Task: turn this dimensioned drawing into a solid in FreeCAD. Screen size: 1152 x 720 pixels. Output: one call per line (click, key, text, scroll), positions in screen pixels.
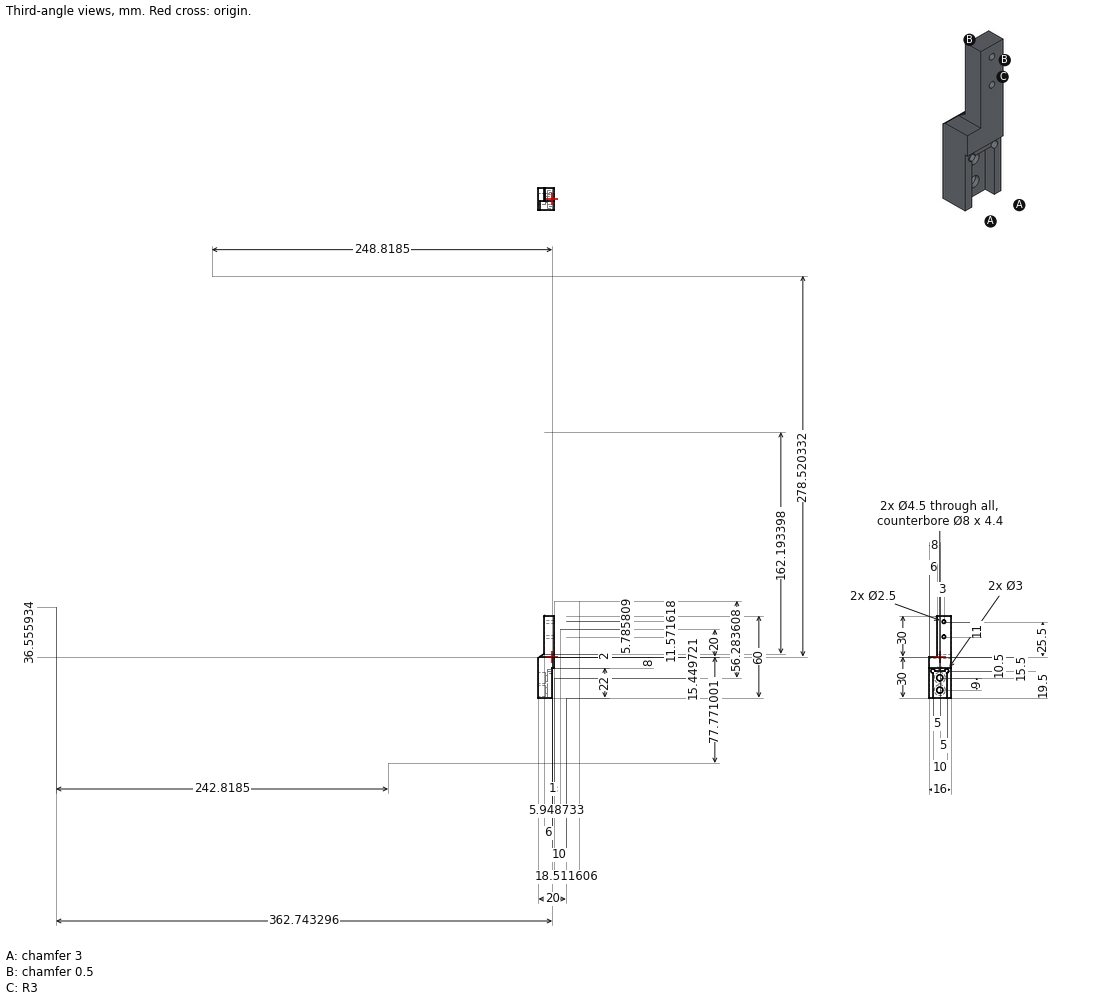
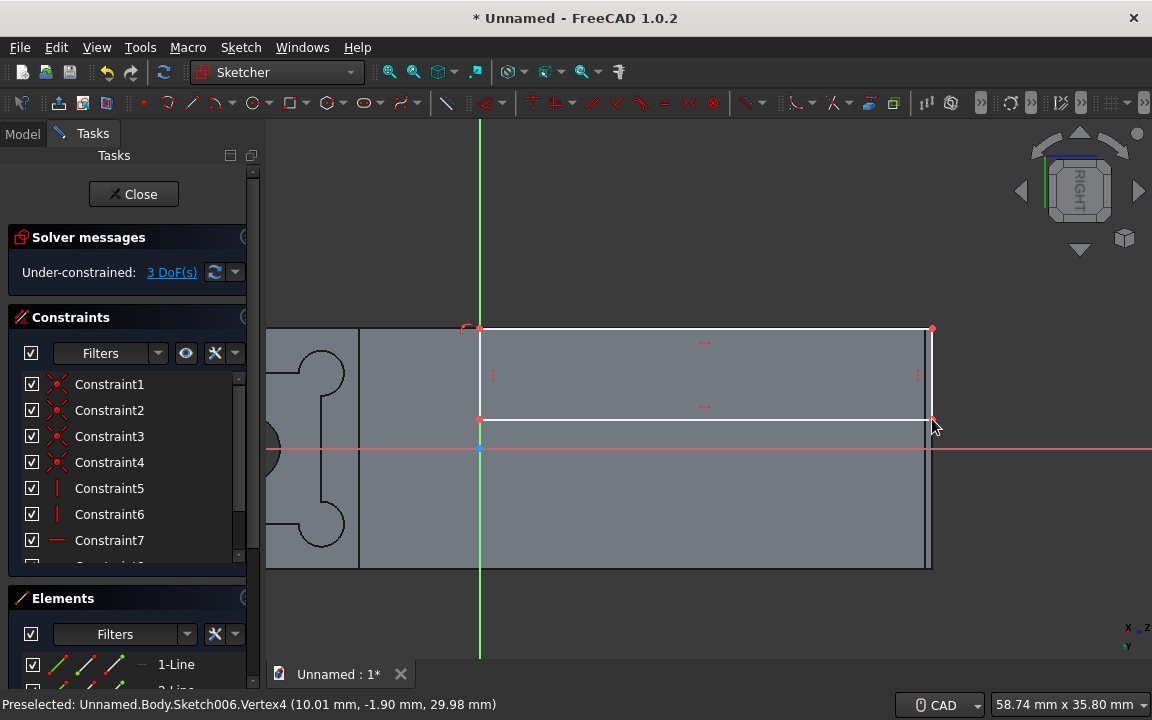
key(d)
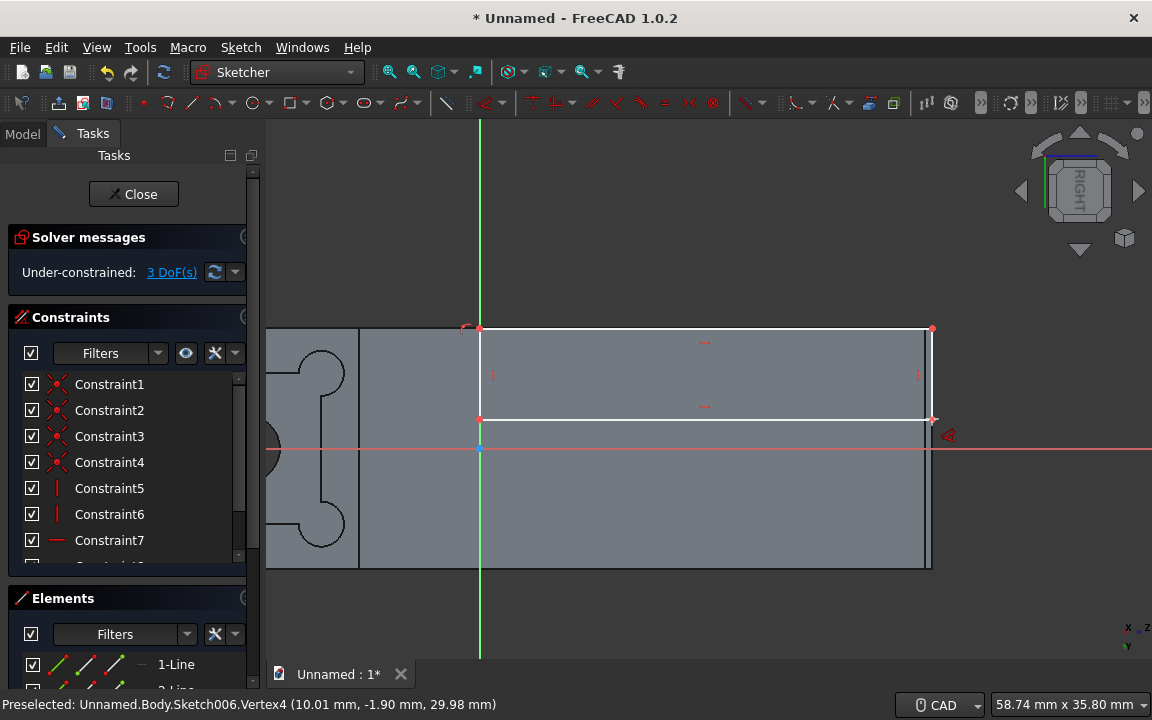
click(480, 356)
click(446, 375)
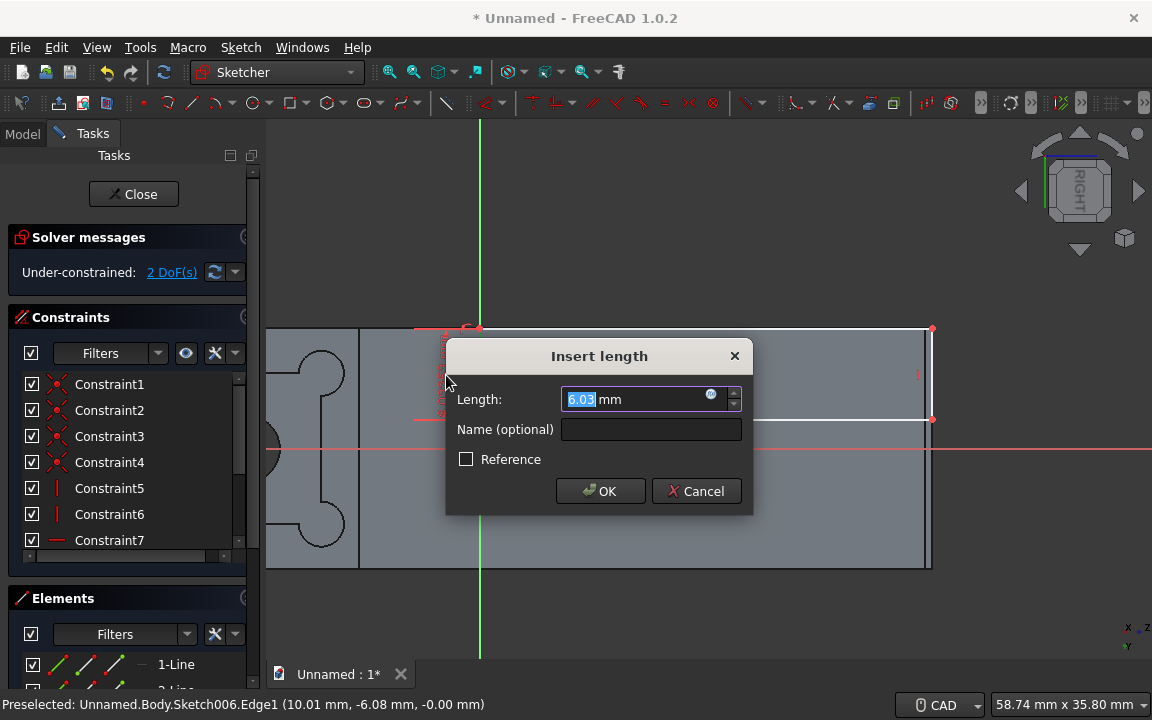
text(6)
key(Return)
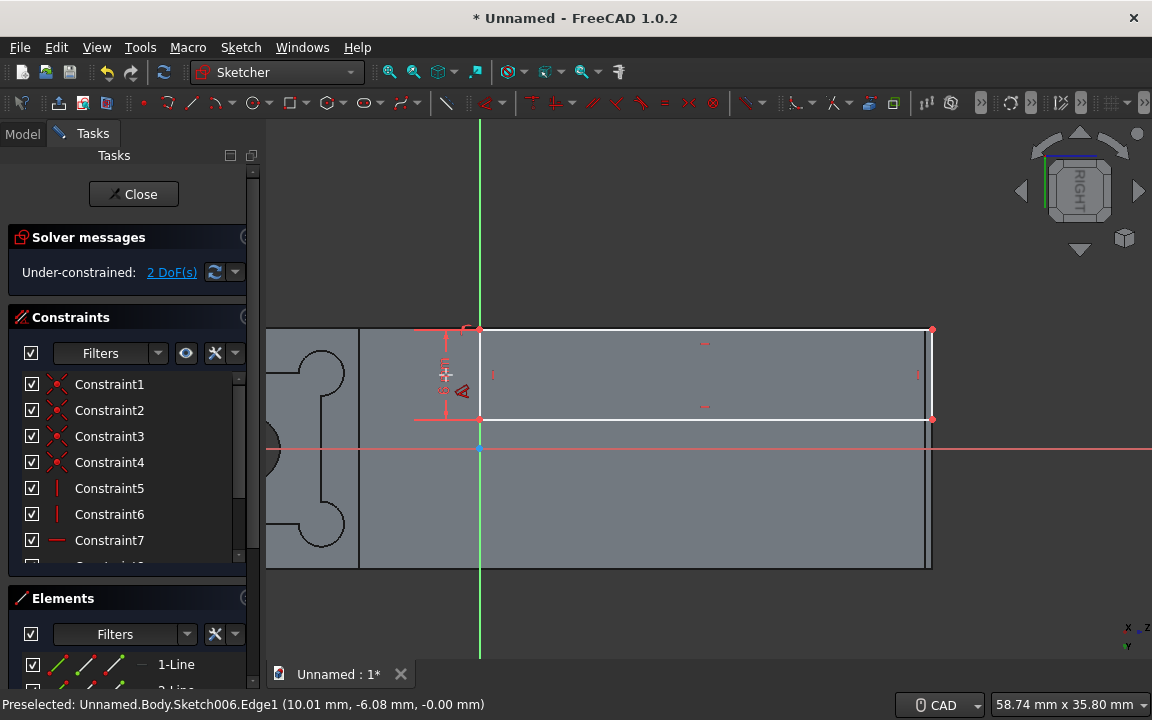
click(615, 420)
click(706, 386)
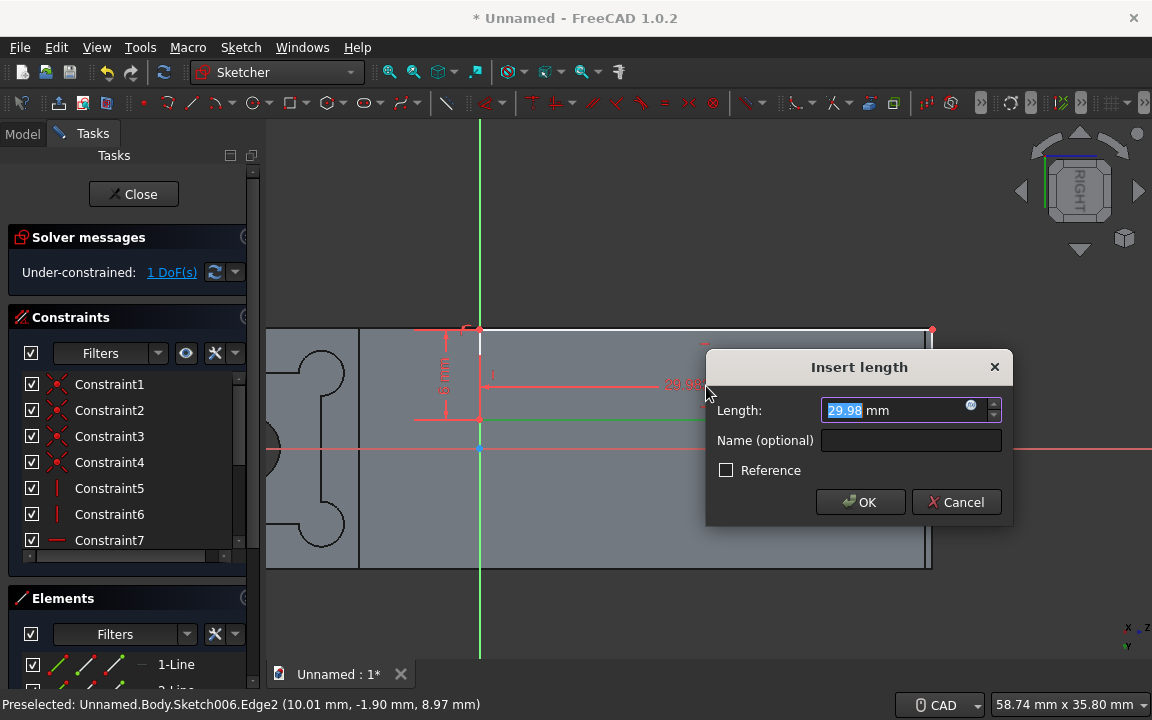
text(30)
key(Return)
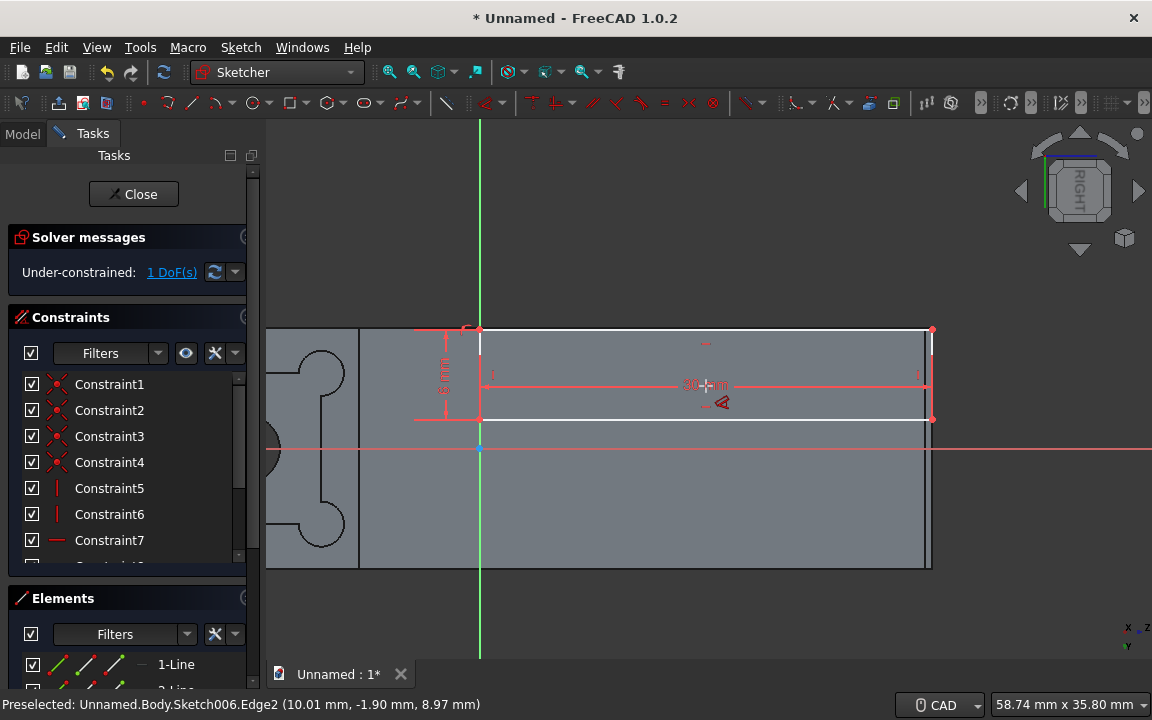
click(480, 330)
click(446, 417)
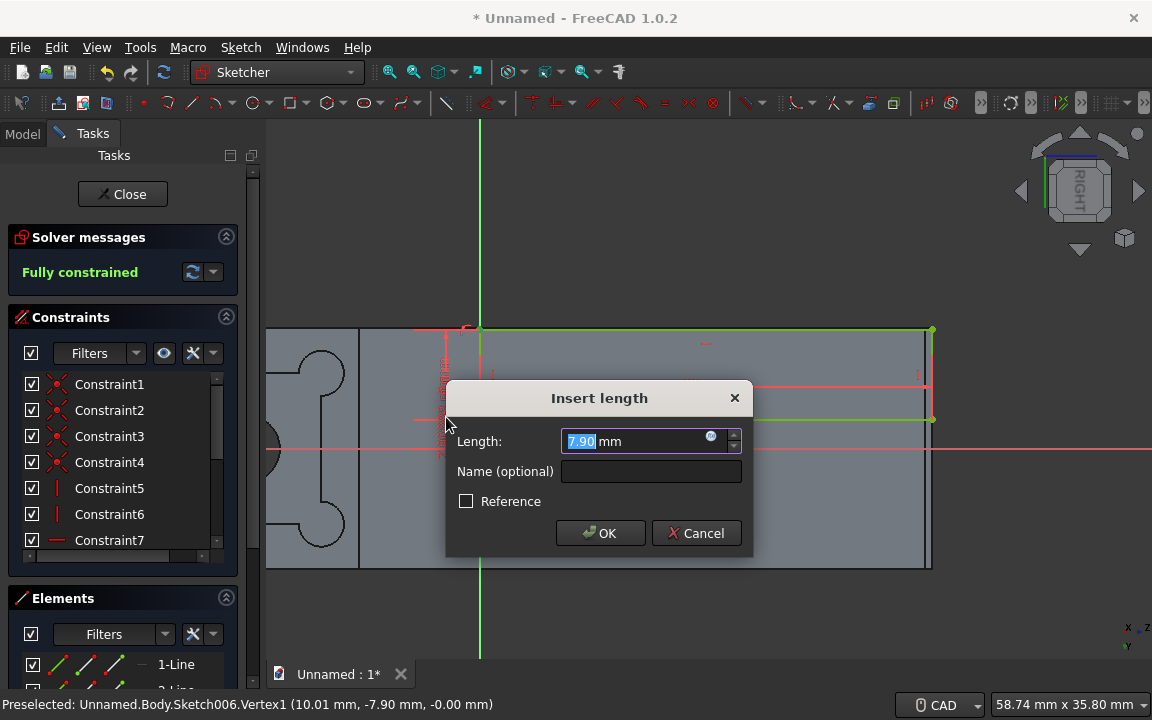
text(8)
key(Return)
key(Escape)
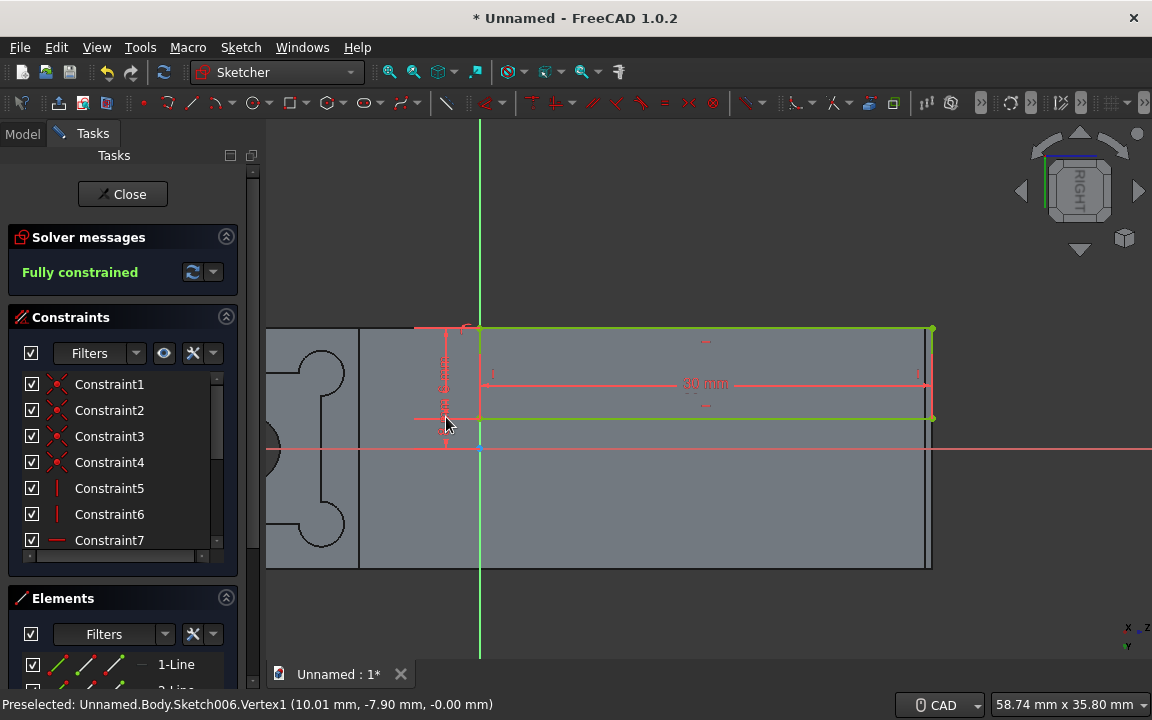
click(123, 194)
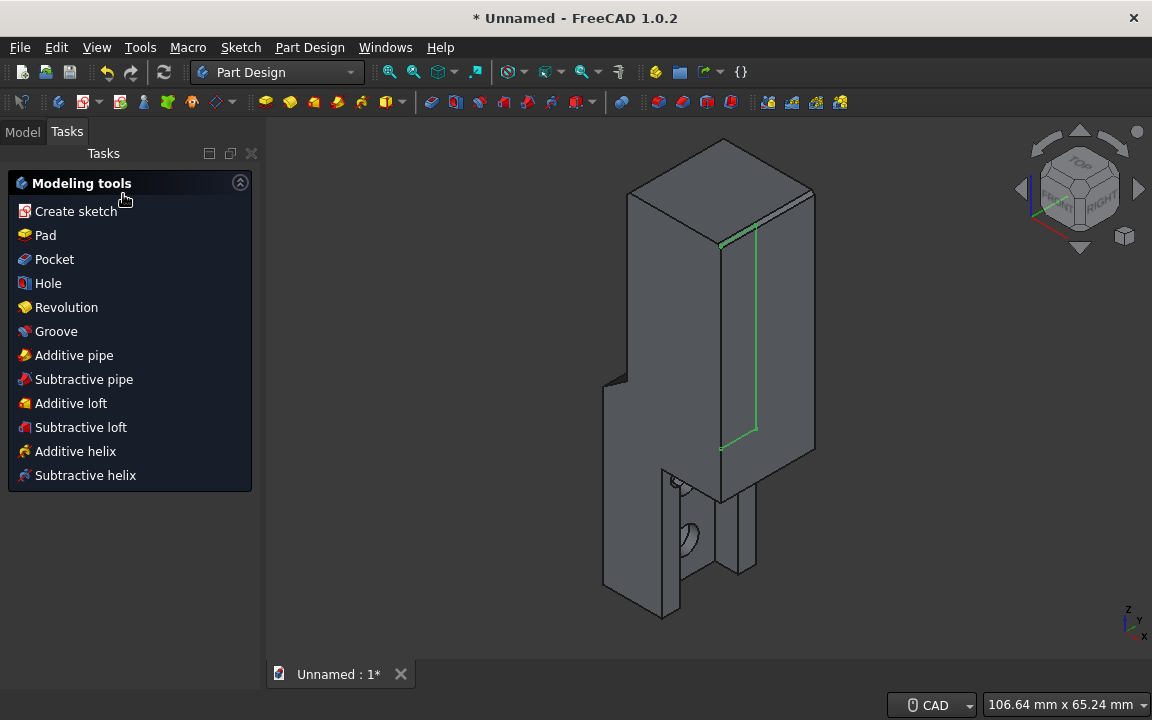
click(432, 102)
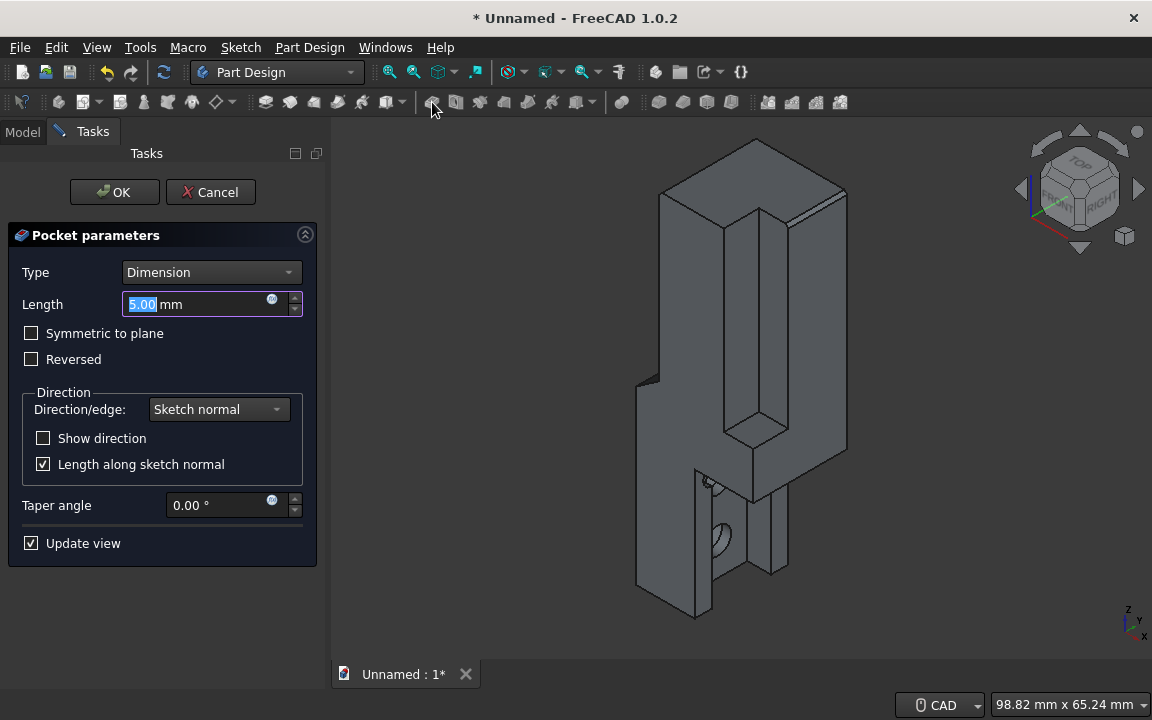
click(212, 272)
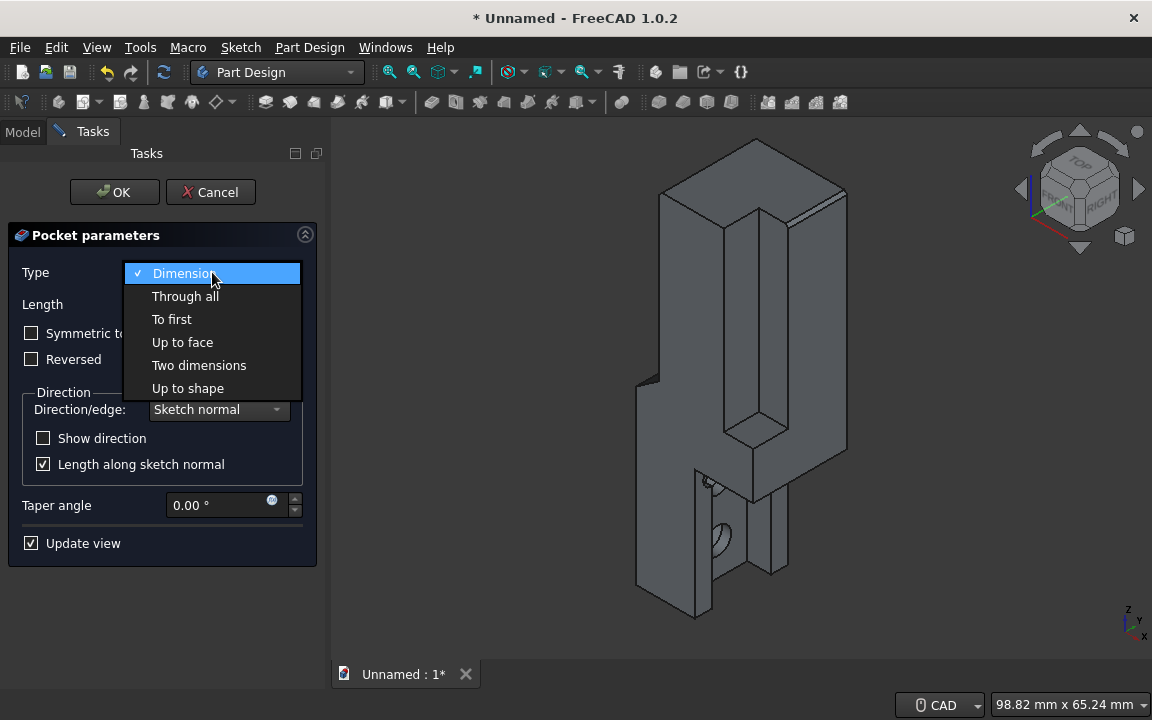
click(212, 296)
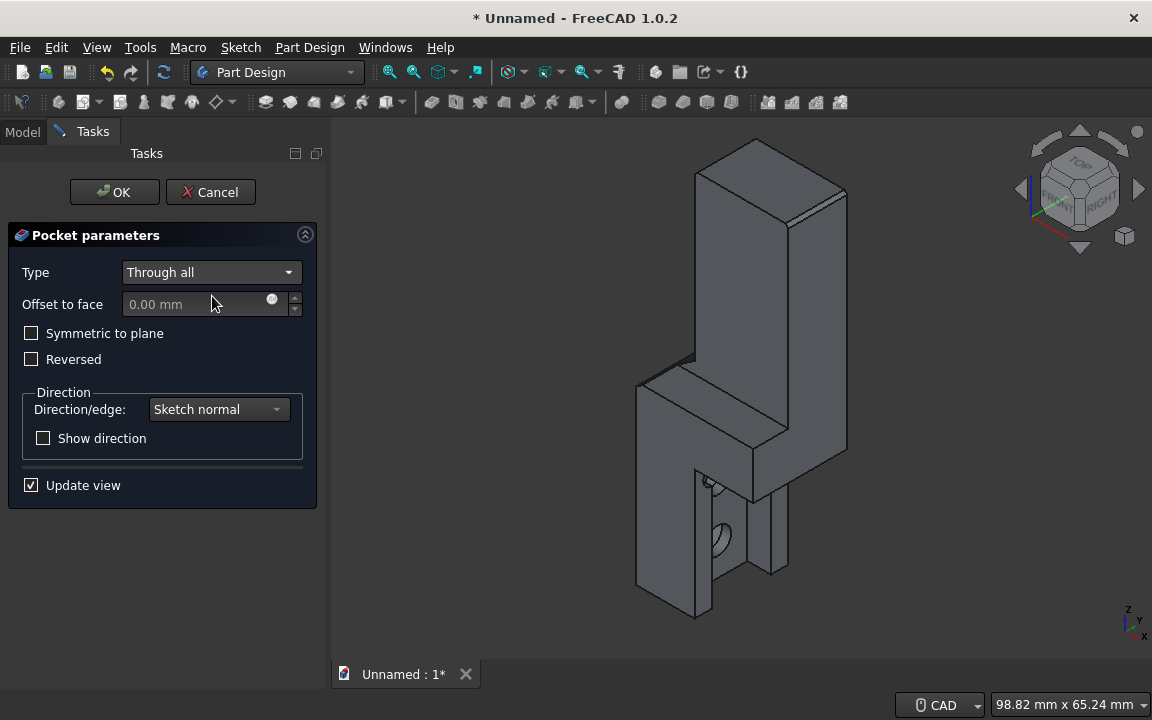
click(115, 192)